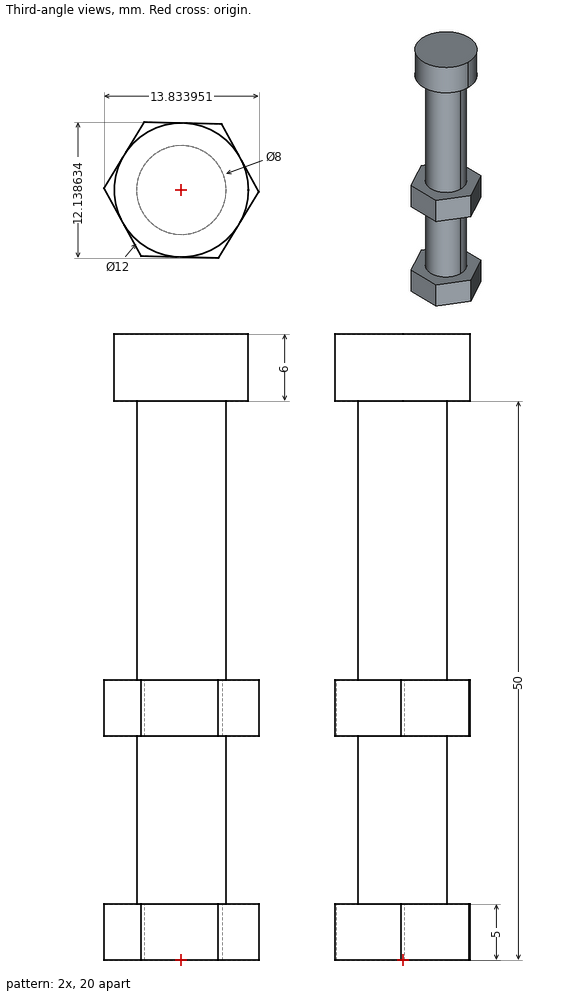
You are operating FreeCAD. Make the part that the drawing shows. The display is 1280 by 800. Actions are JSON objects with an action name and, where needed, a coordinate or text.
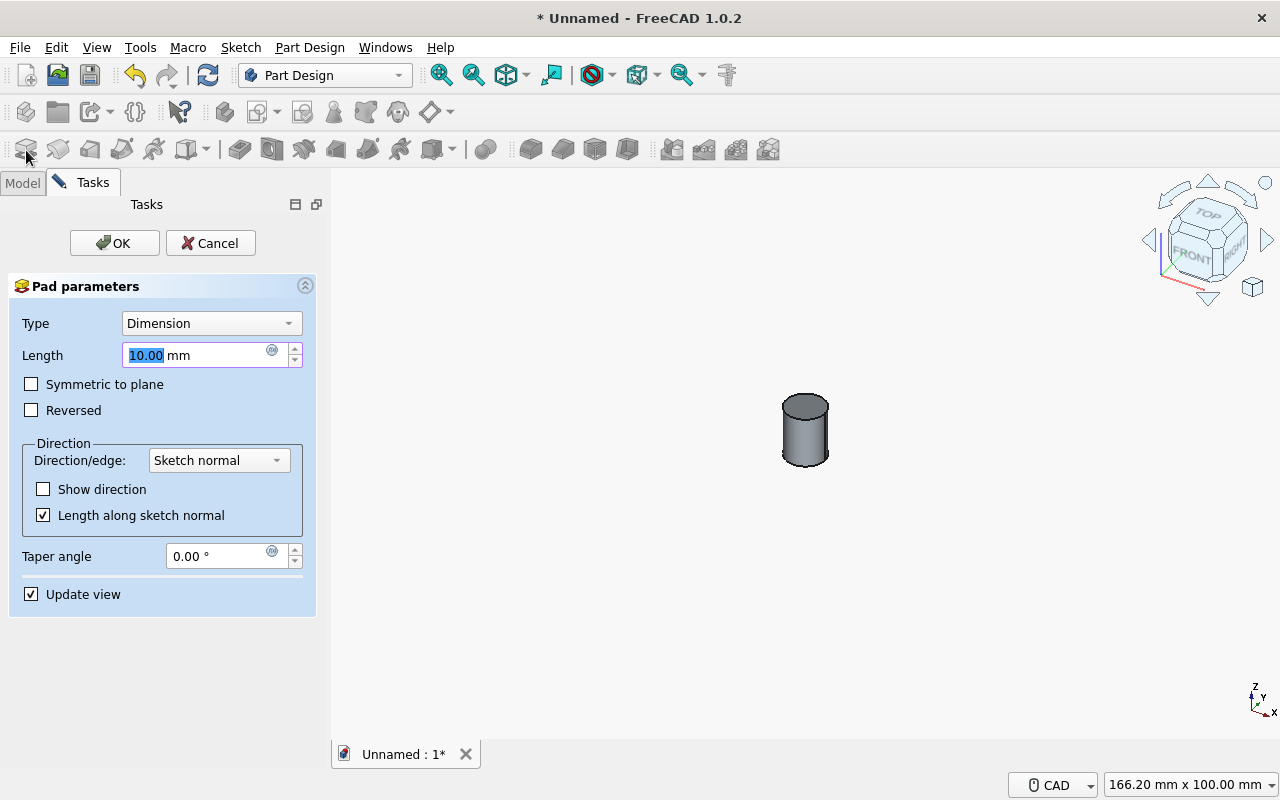
{"action": "type", "text": "50"}
{"action": "key", "text": "Tab"}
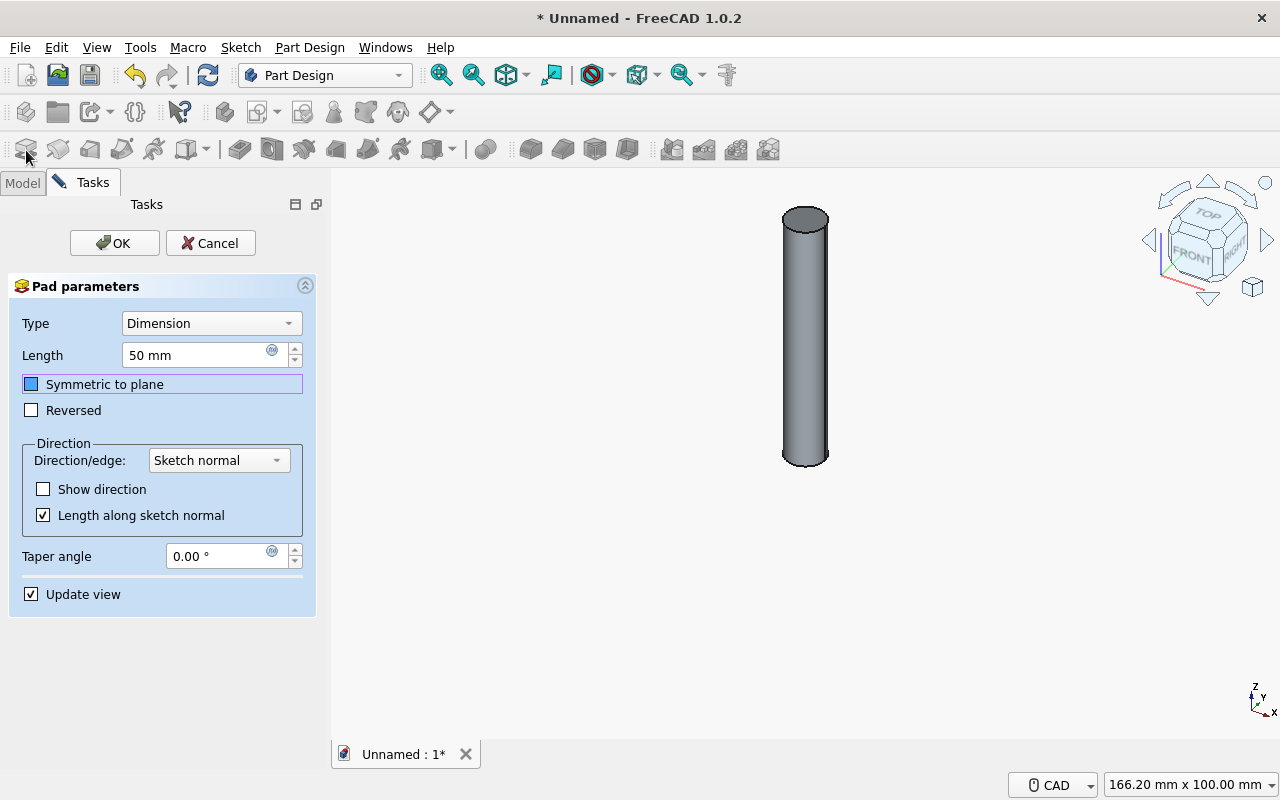
{"action": "left_click", "coordinate": [115, 243]}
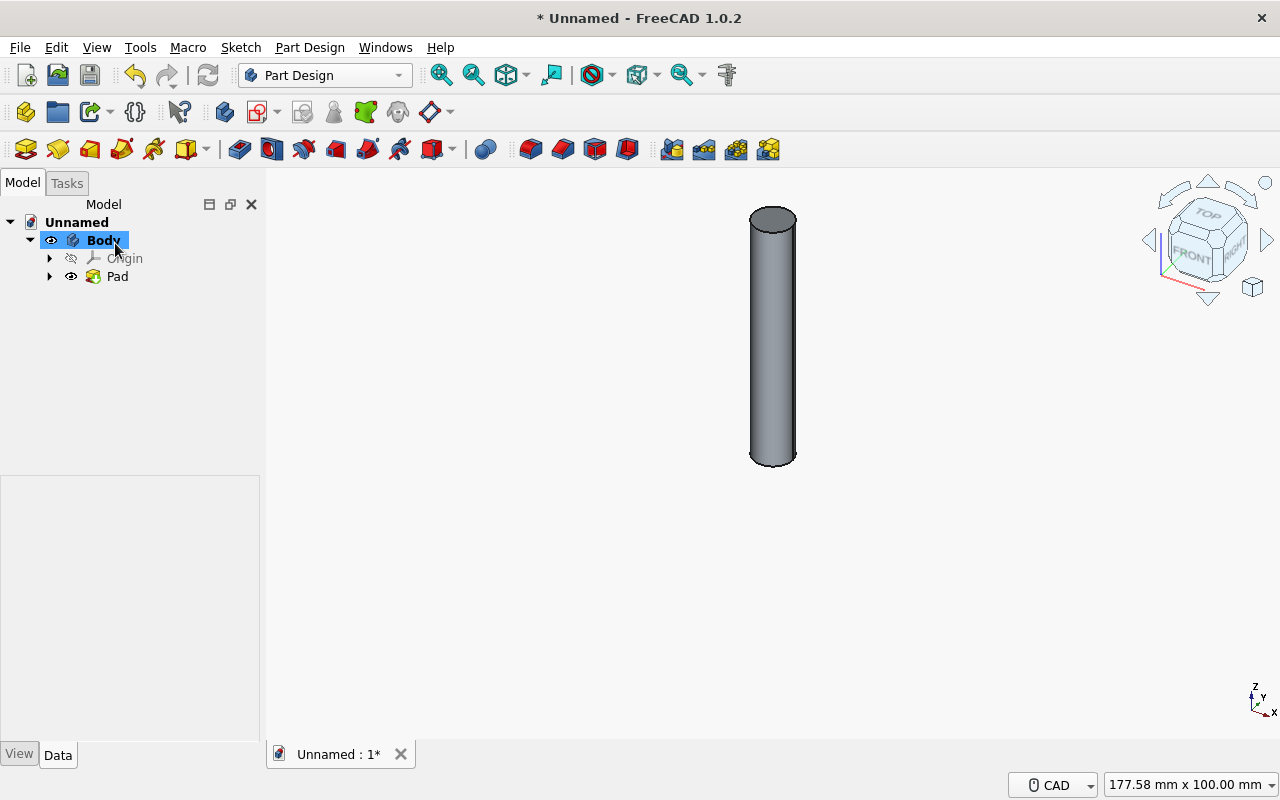
{"action": "left_click", "coordinate": [773, 219]}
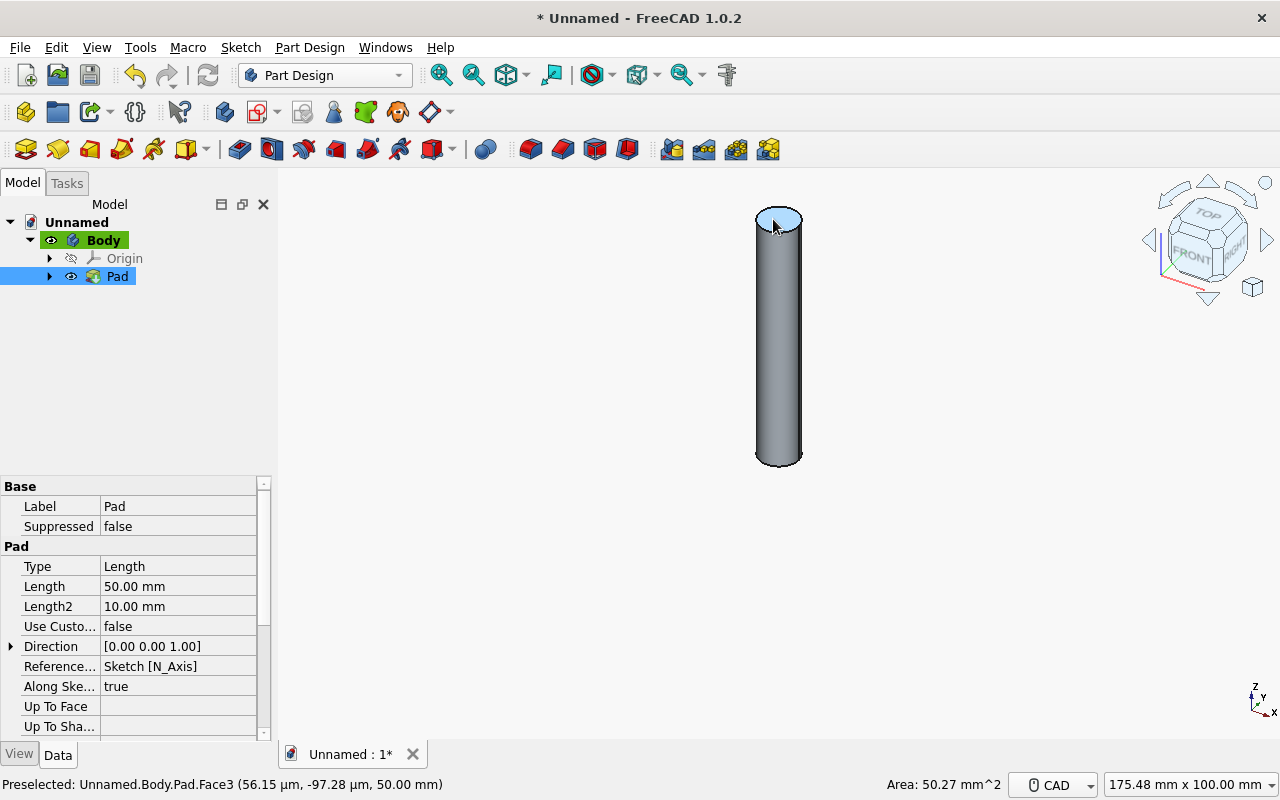
{"action": "left_click", "coordinate": [258, 112]}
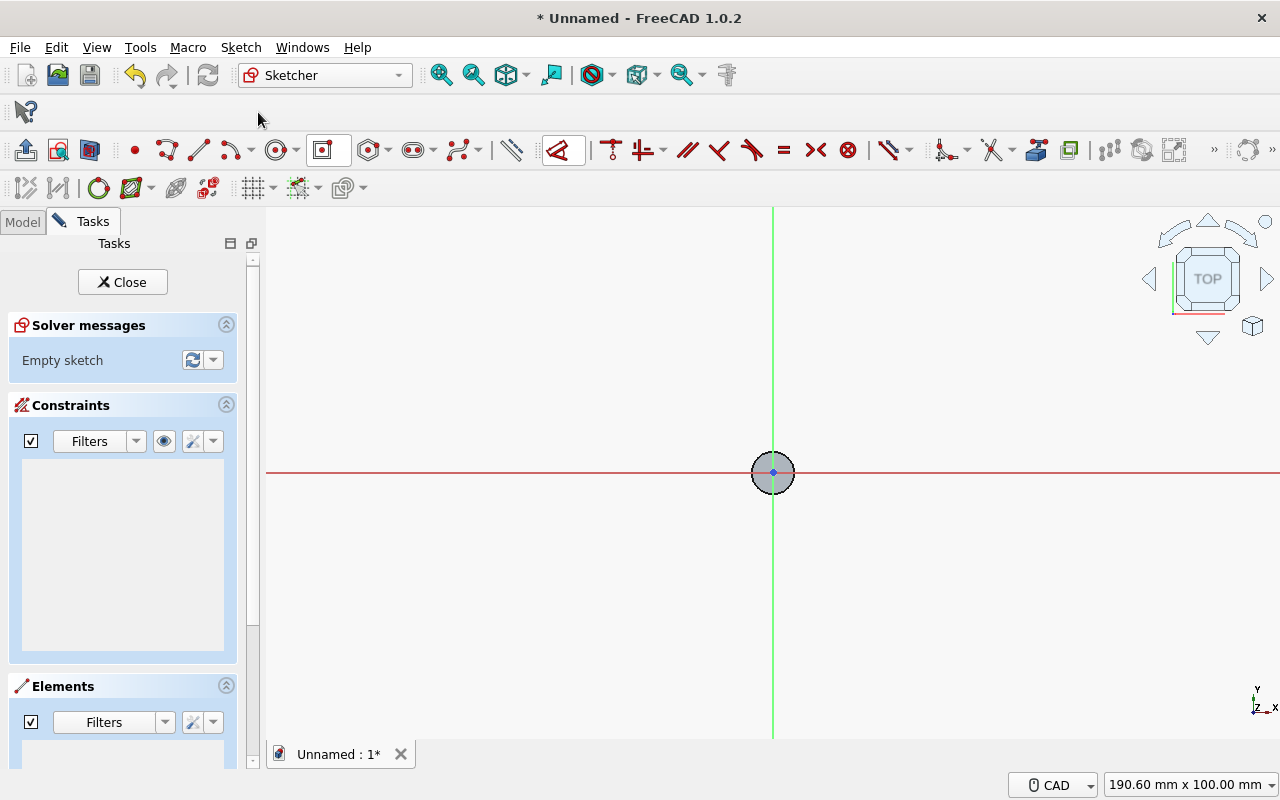
{"action": "scroll", "coordinate": [790, 473], "scroll_direction": "up", "scroll_amount": 8}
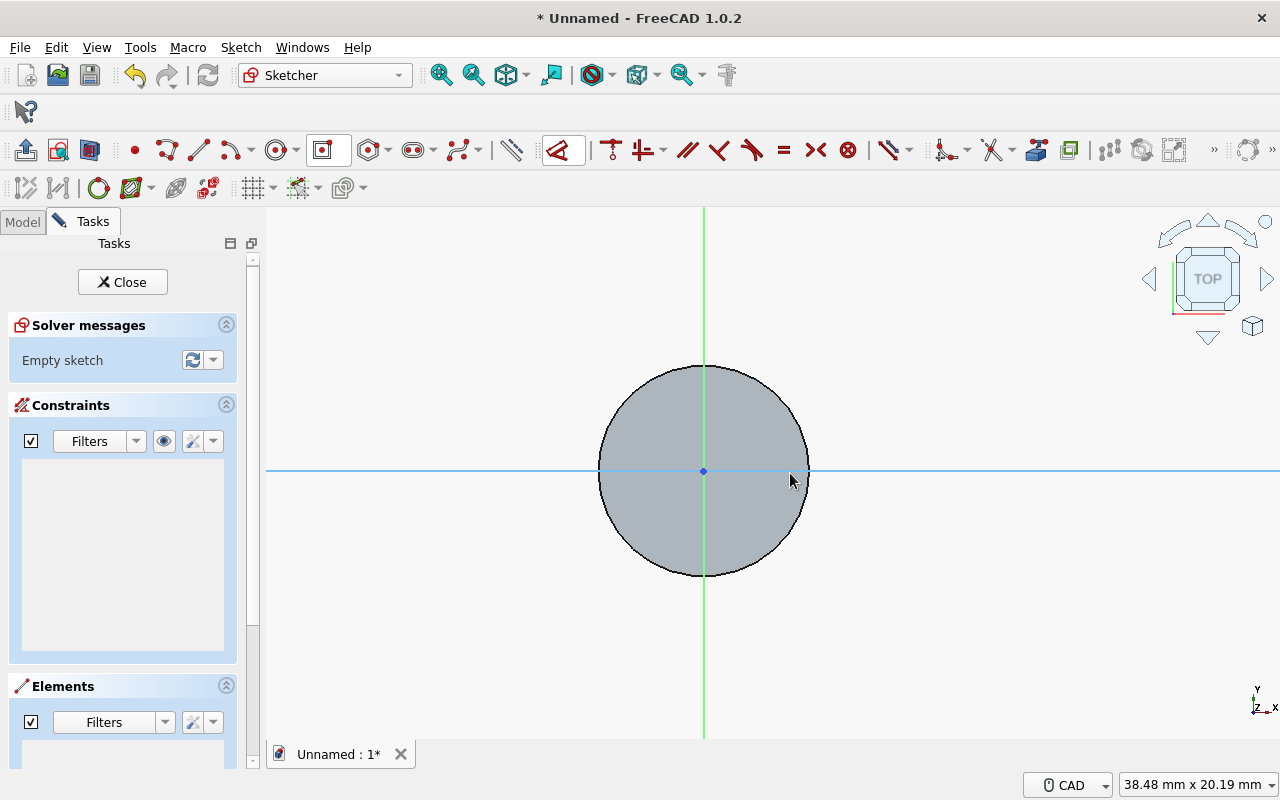
{"action": "left_click", "coordinate": [276, 150]}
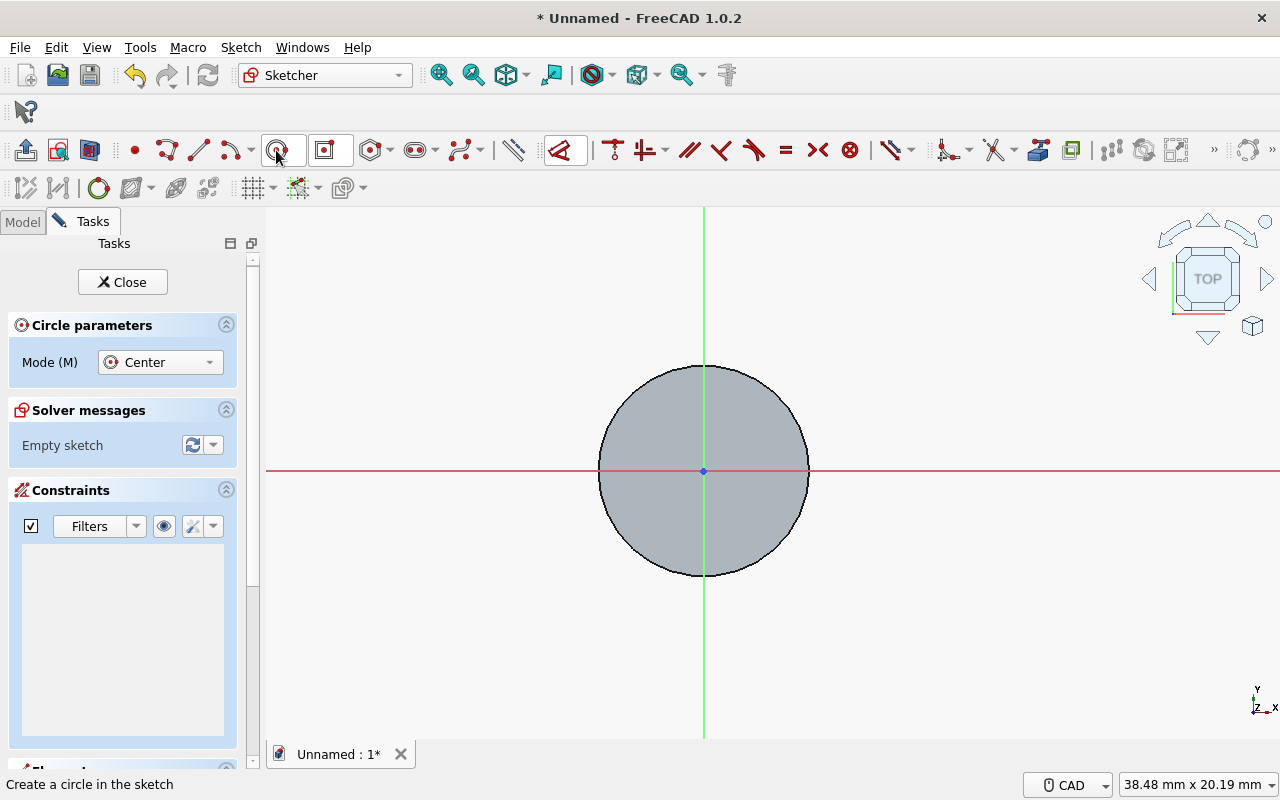
{"action": "left_click", "coordinate": [704, 471]}
{"action": "mouse_move", "coordinate": [816, 359]}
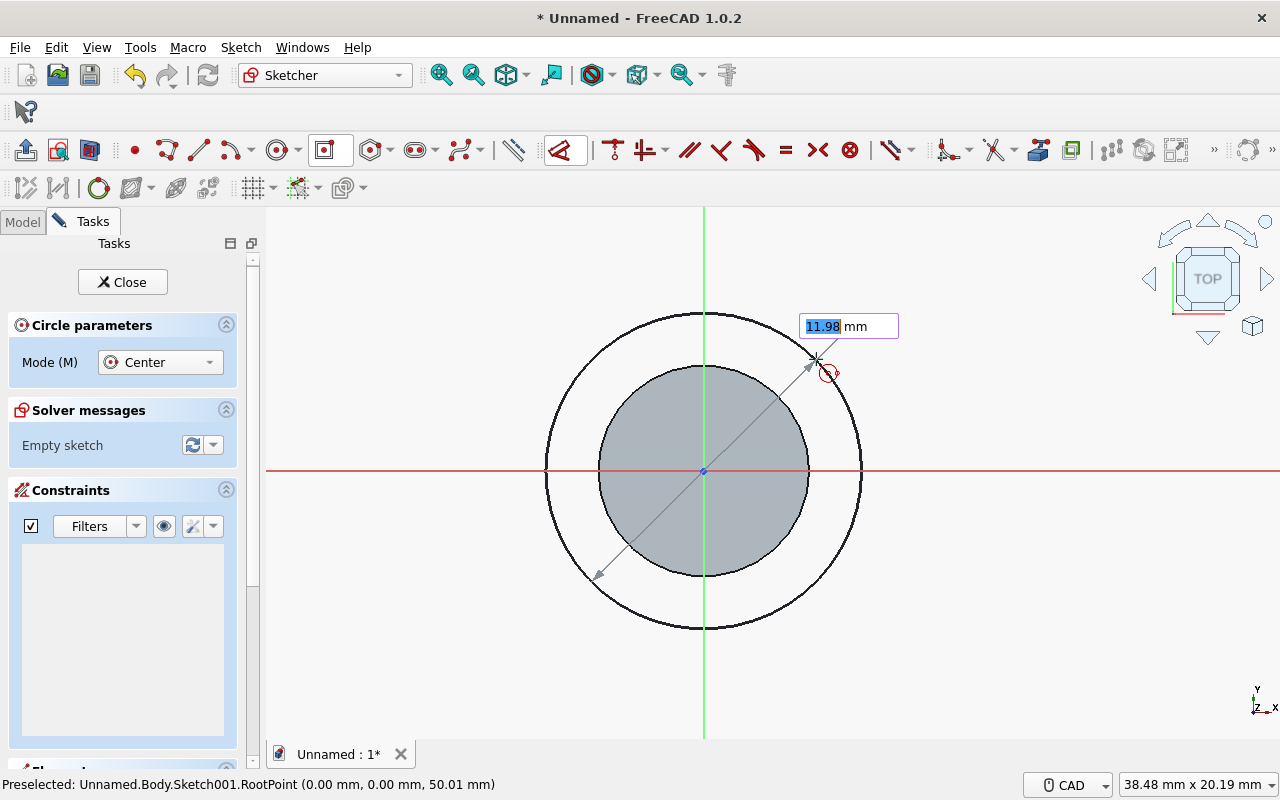
{"action": "type", "text": "12"}
{"action": "key", "text": "Return"}
{"action": "key", "text": "Escape"}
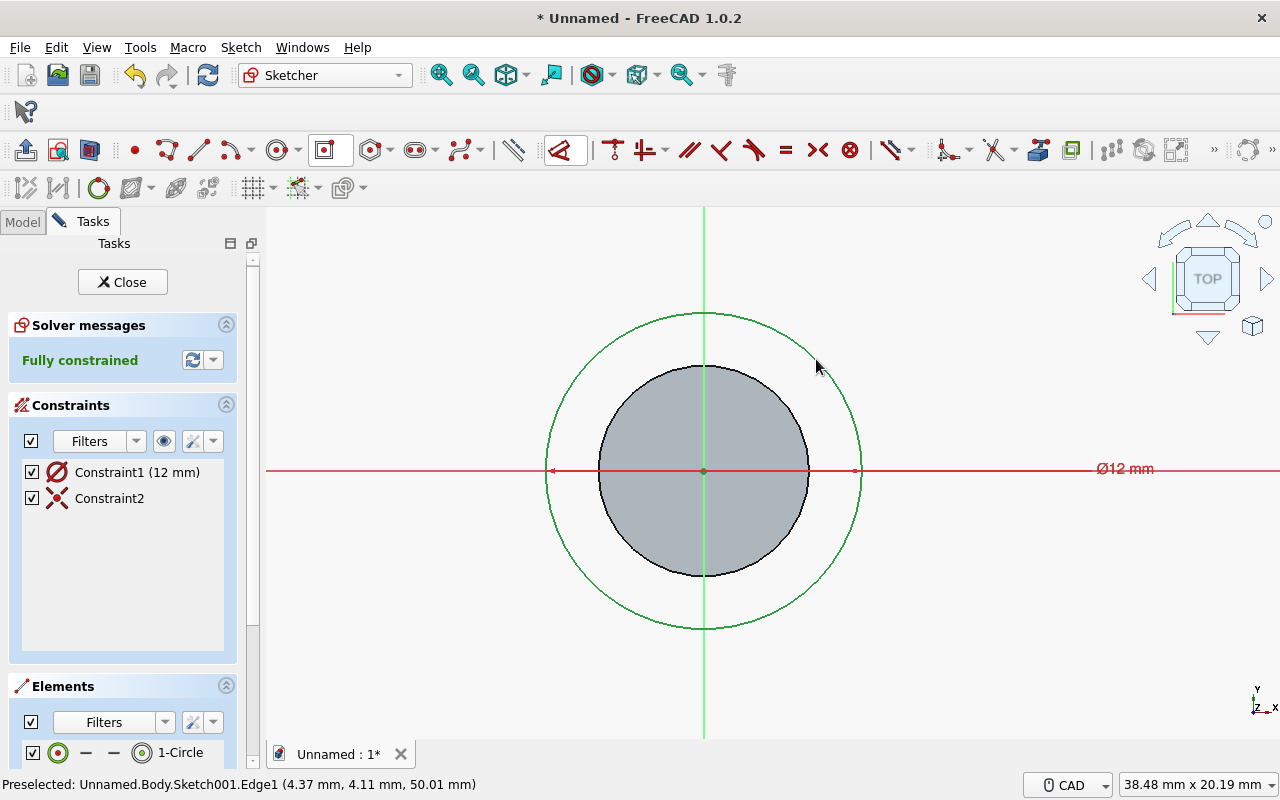
{"action": "left_click", "coordinate": [123, 282]}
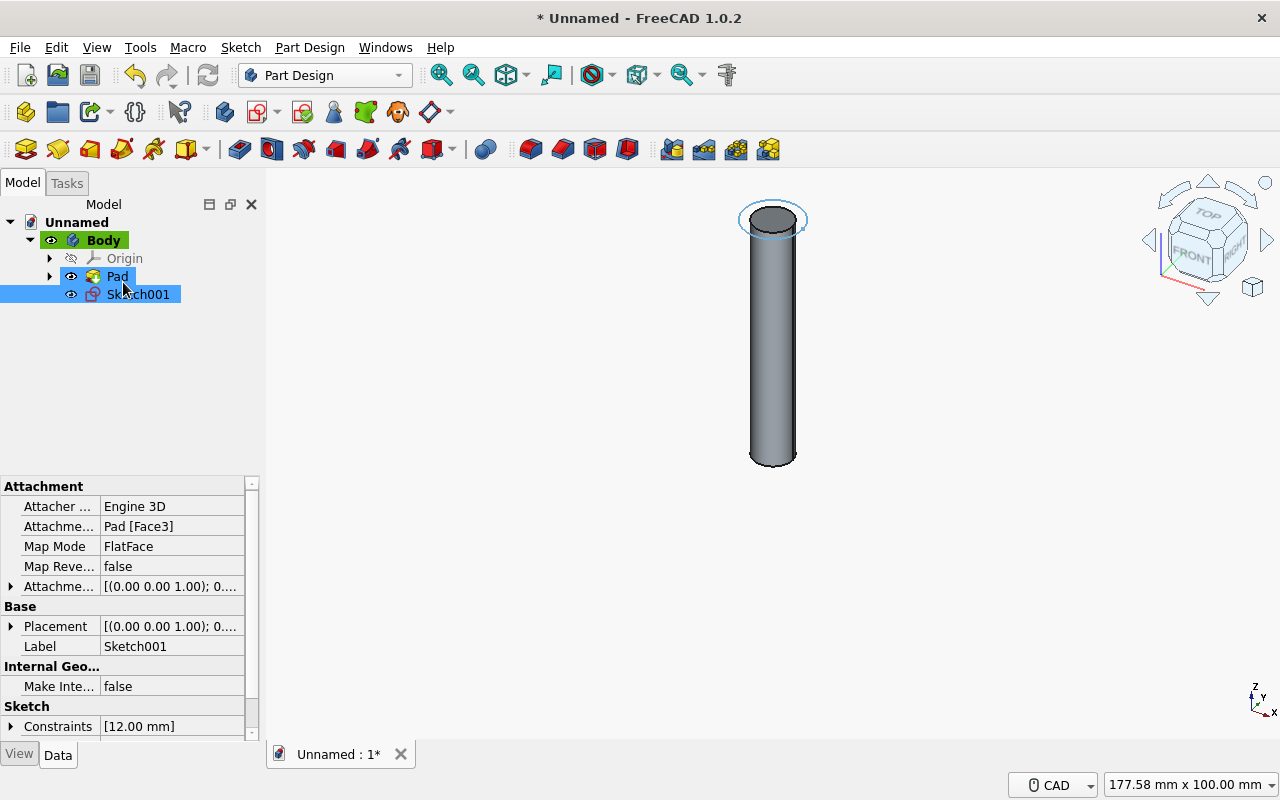
{"action": "left_click", "coordinate": [26, 150]}